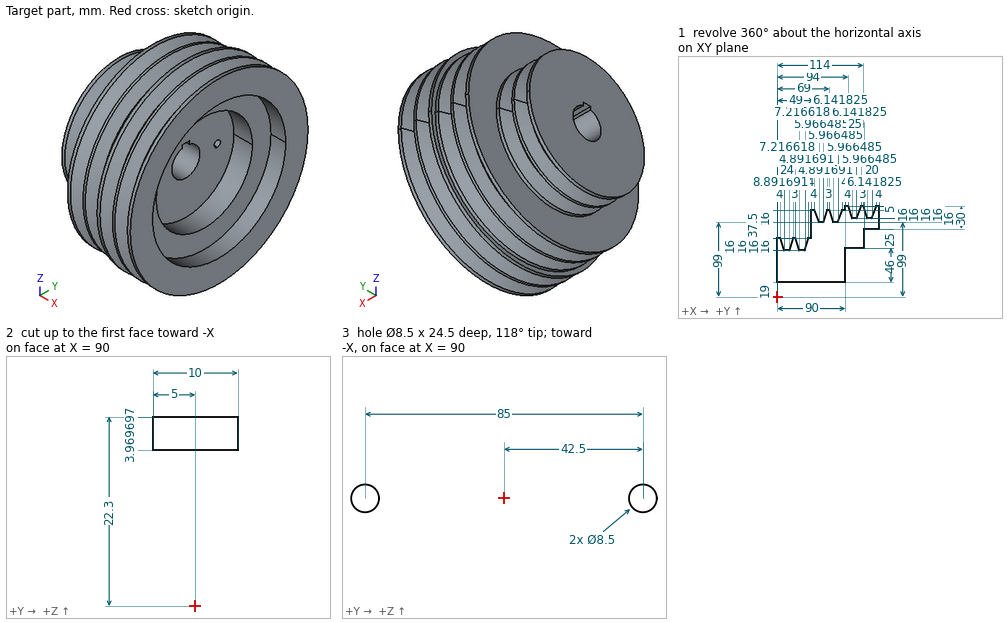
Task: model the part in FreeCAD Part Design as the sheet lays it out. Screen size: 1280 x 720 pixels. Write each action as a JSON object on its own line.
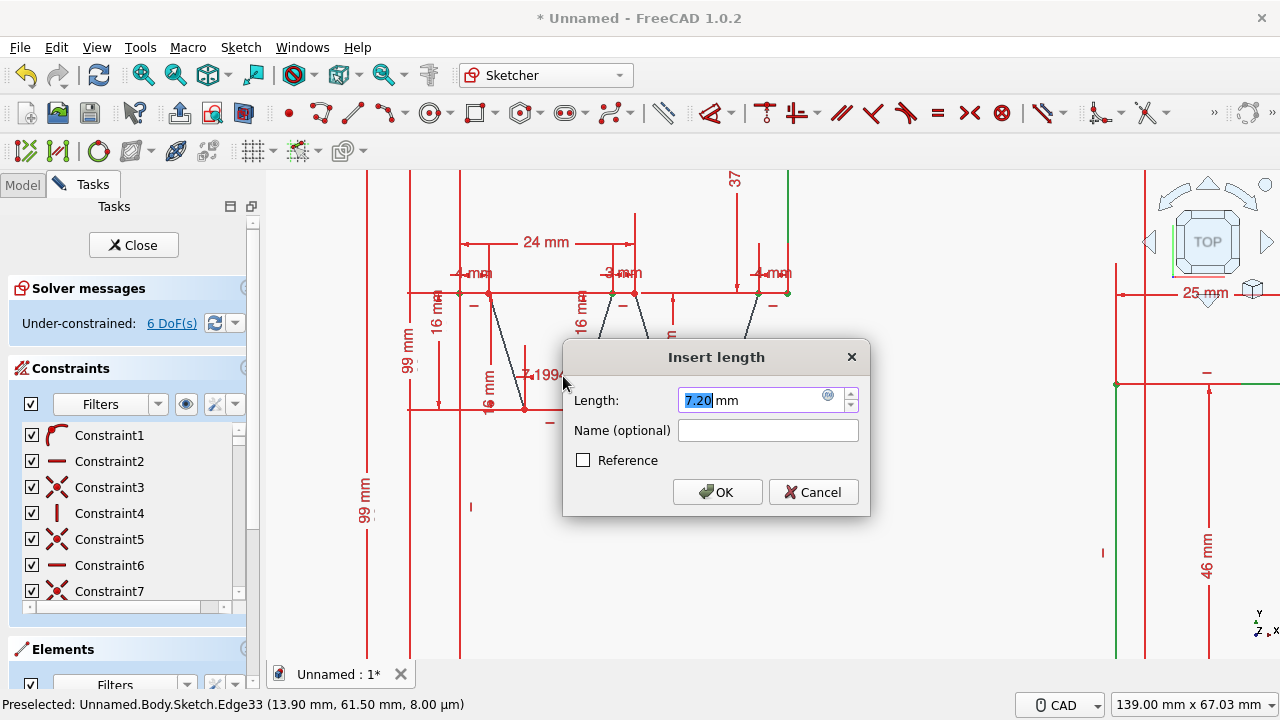
{"action": "type", "text": "7.216618"}
{"action": "key", "text": "Return"}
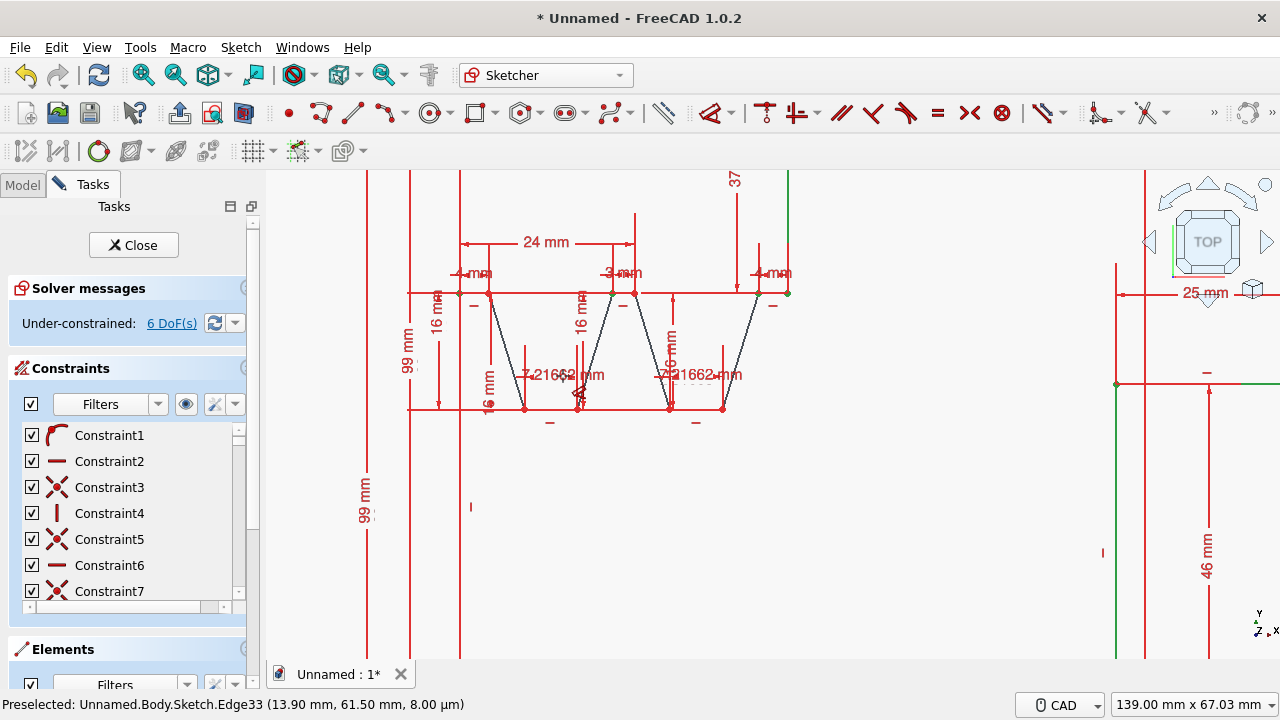
{"action": "left_click", "coordinate": [525, 410]}
{"action": "left_click", "coordinate": [492, 352]}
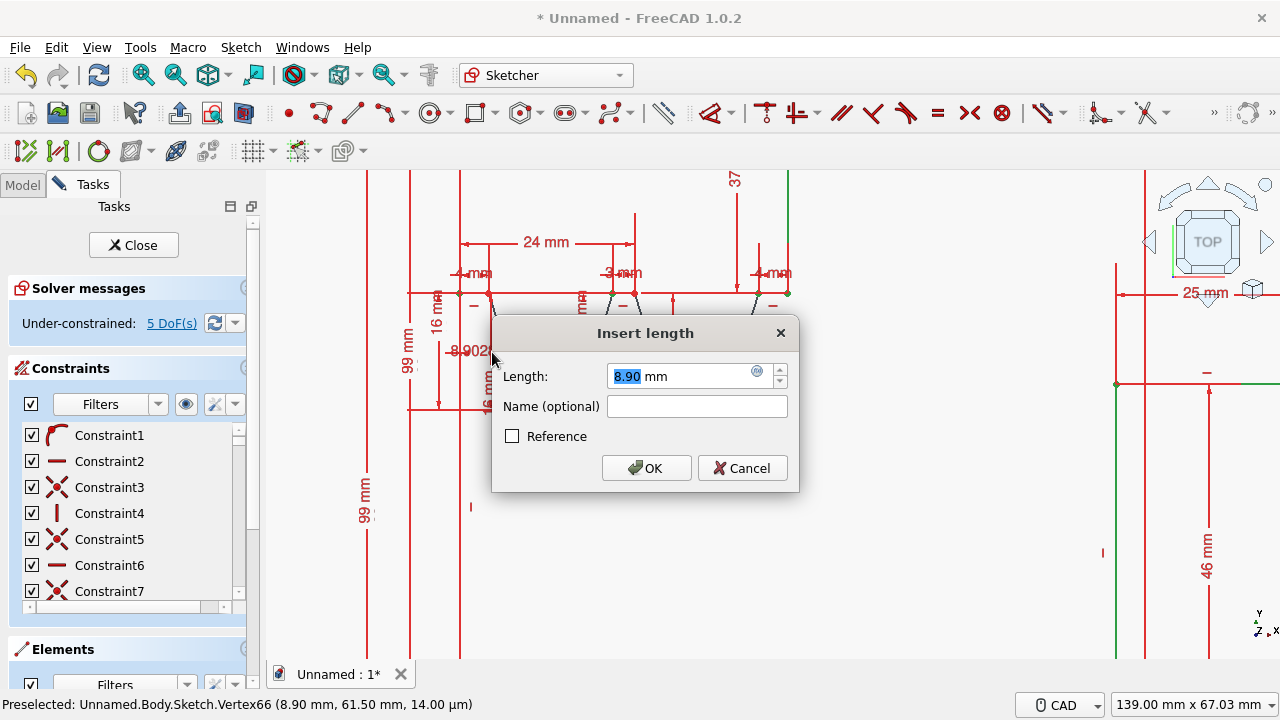
{"action": "type", "text": "8.891691"}
{"action": "key", "text": "Return"}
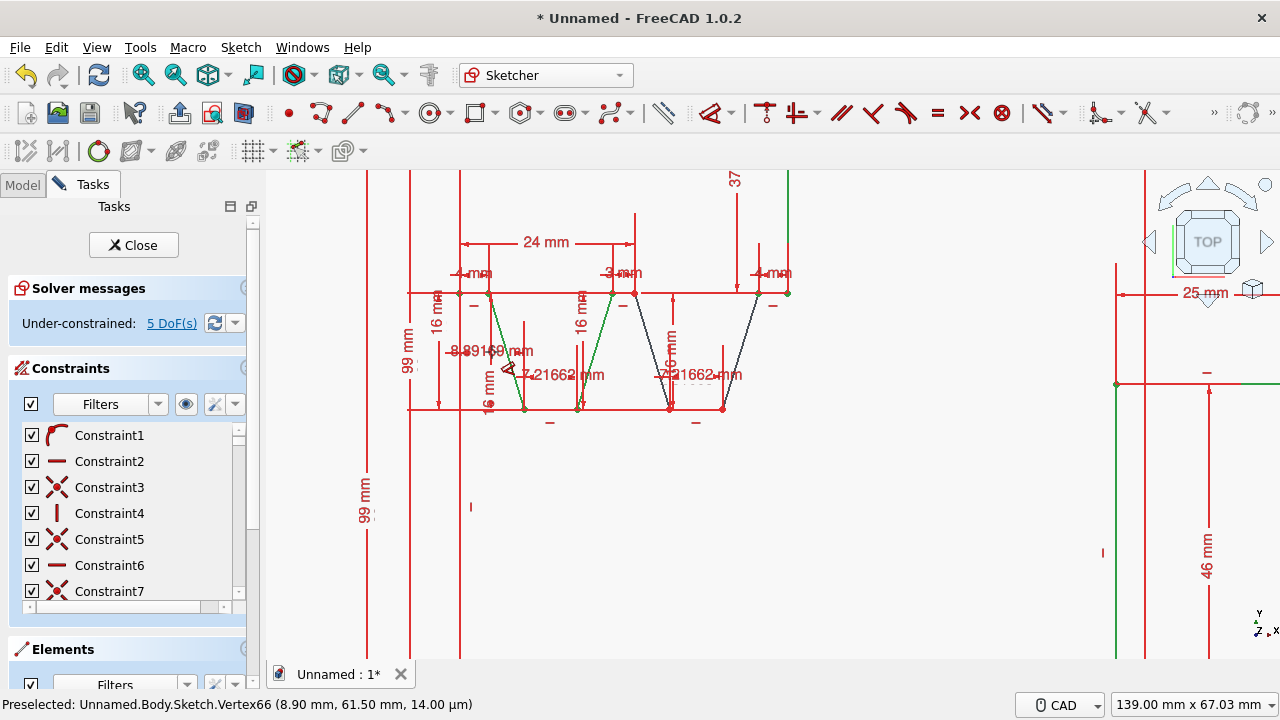
{"action": "scroll", "coordinate": [560, 411], "scroll_direction": "down", "scroll_amount": 5}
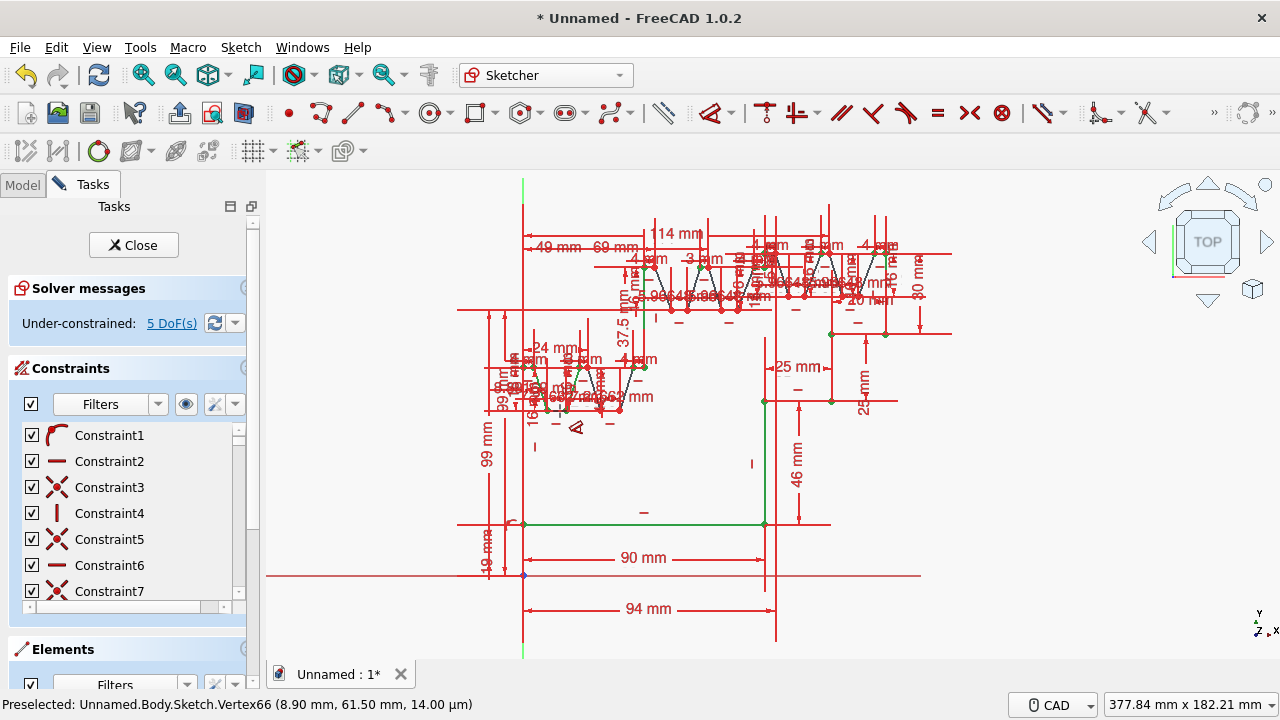
{"action": "scroll", "coordinate": [870, 267], "scroll_direction": "up", "scroll_amount": 5}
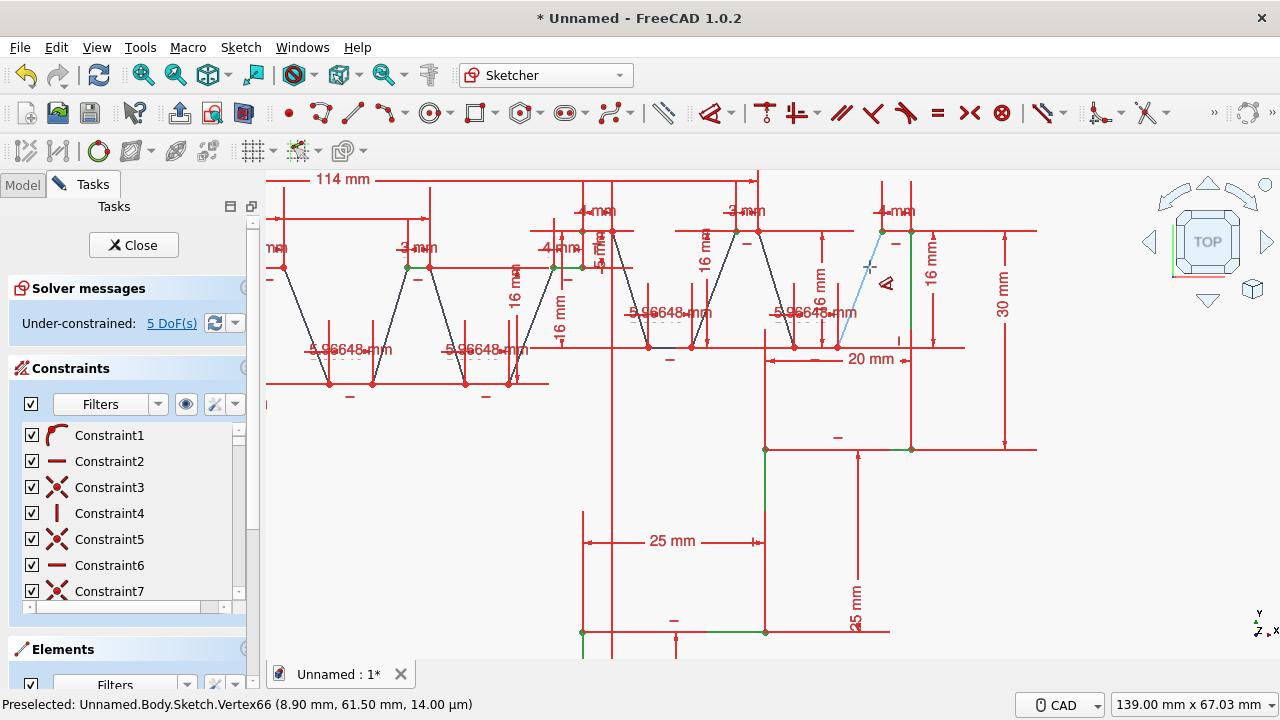
{"action": "left_click", "coordinate": [869, 266]}
{"action": "left_click", "coordinate": [860, 382]}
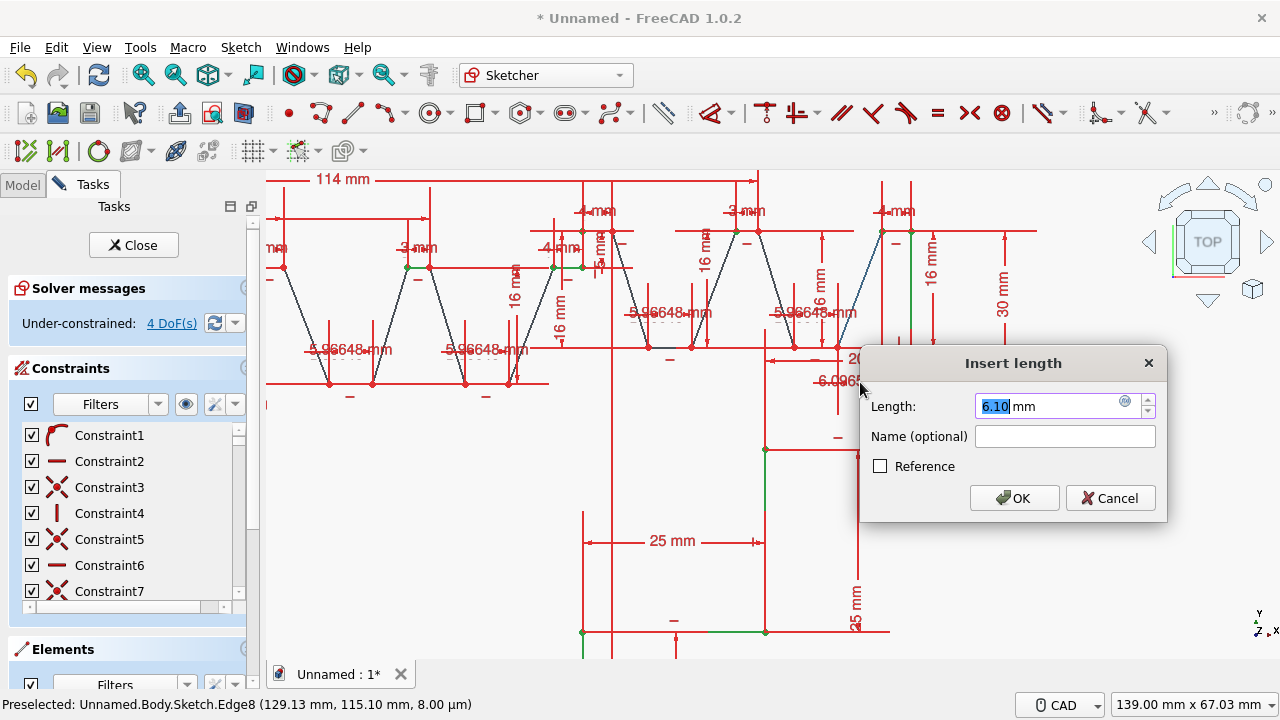
{"action": "type", "text": "6.141825"}
{"action": "key", "text": "Return"}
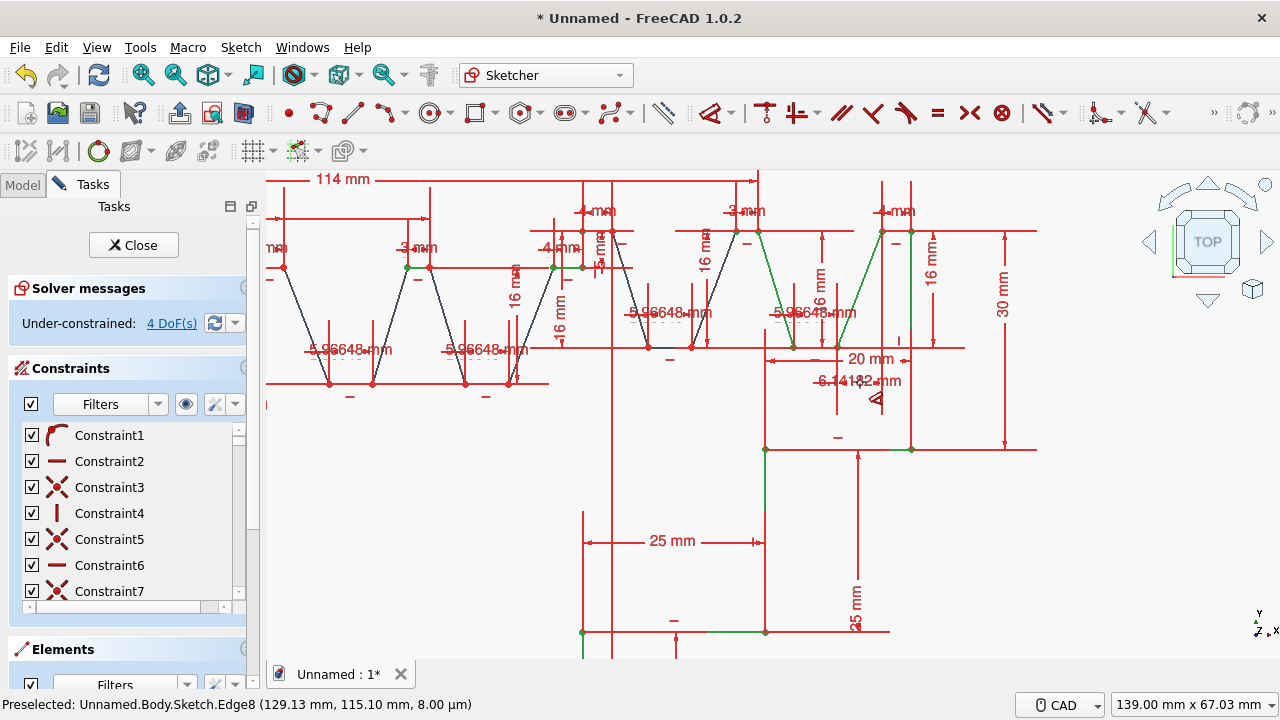
{"action": "left_click", "coordinate": [723, 266]}
{"action": "left_click", "coordinate": [714, 382]}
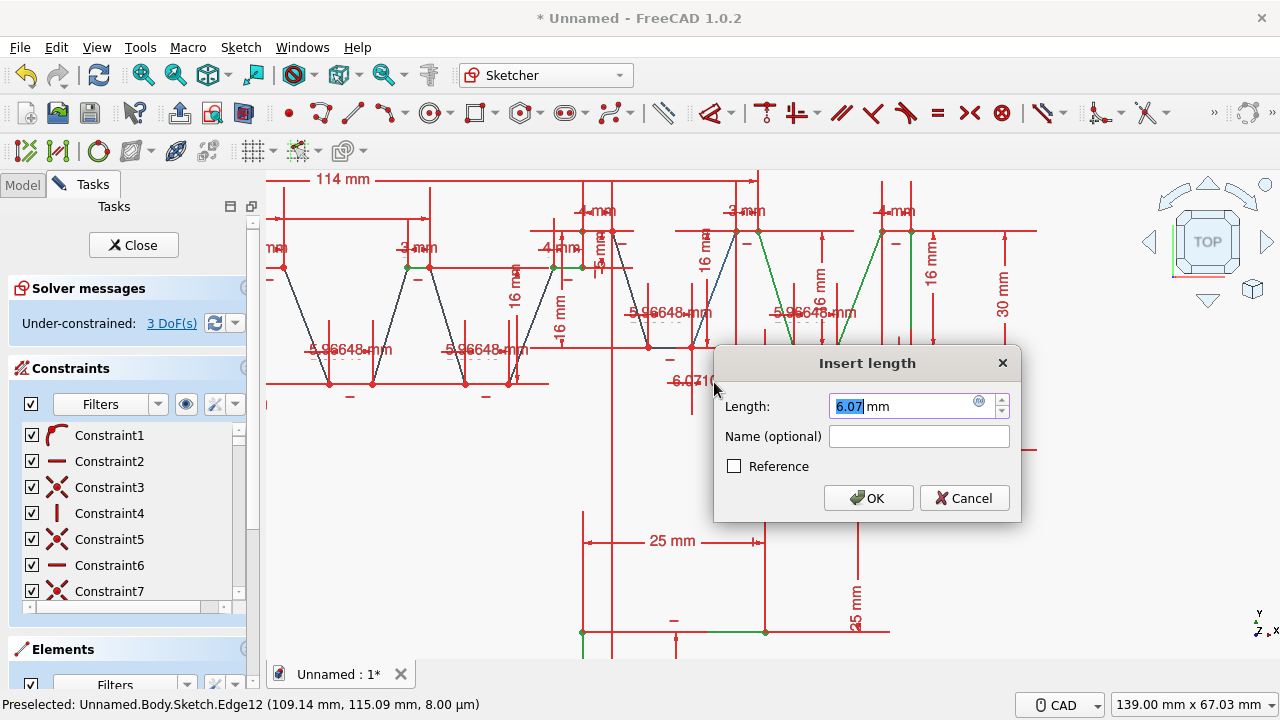
{"action": "type", "text": "6.141825"}
{"action": "key", "text": "Return"}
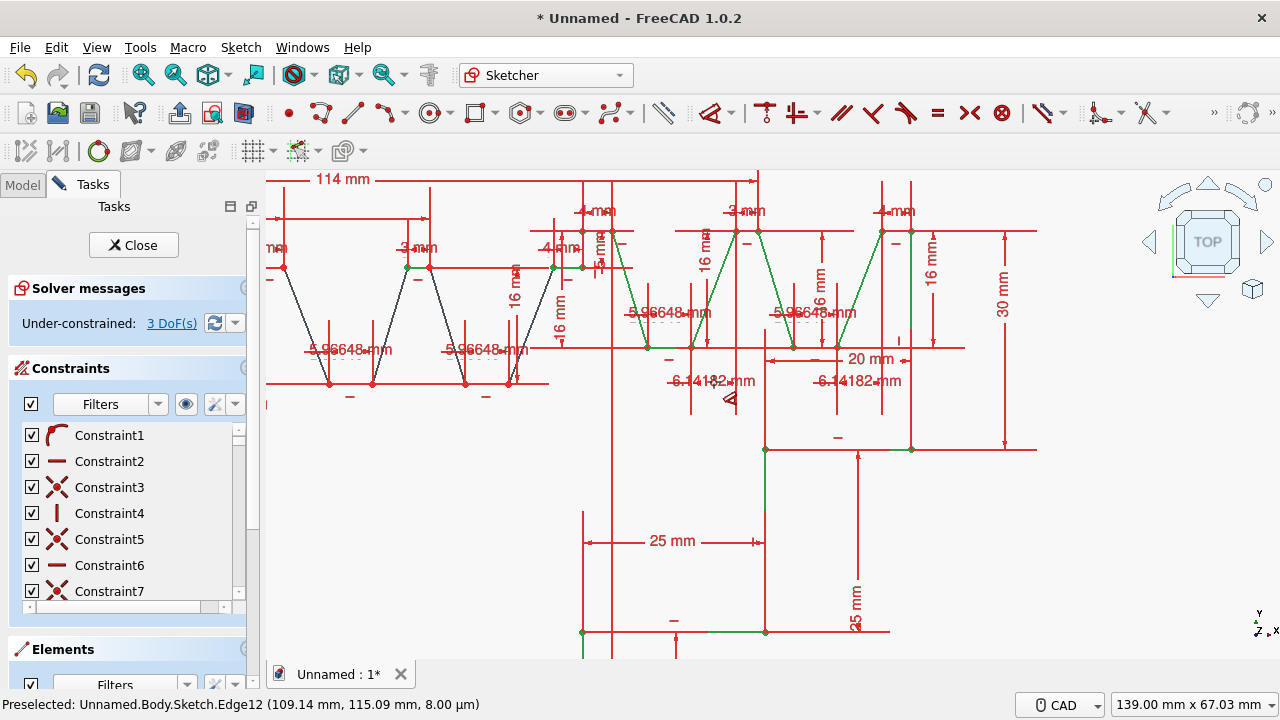
{"action": "left_click", "coordinate": [540, 303]}
{"action": "left_click", "coordinate": [531, 418]}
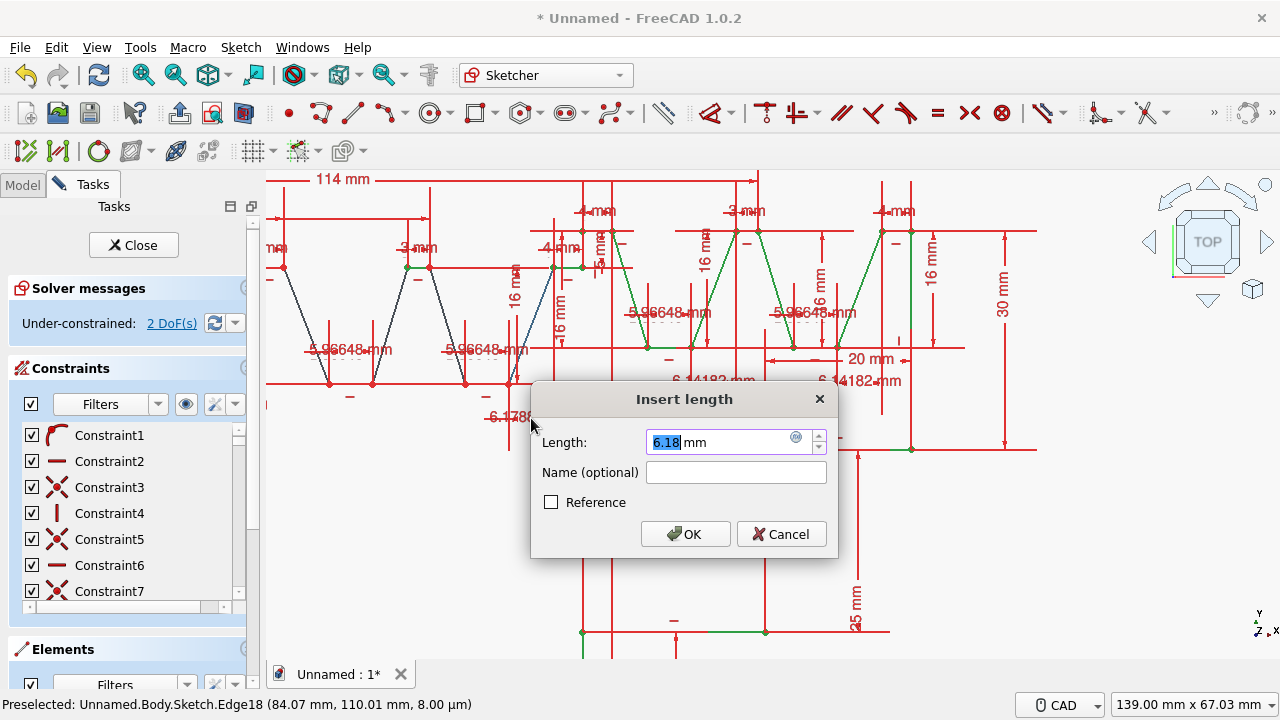
{"action": "type", "text": "6.141825"}
{"action": "key", "text": "Return"}